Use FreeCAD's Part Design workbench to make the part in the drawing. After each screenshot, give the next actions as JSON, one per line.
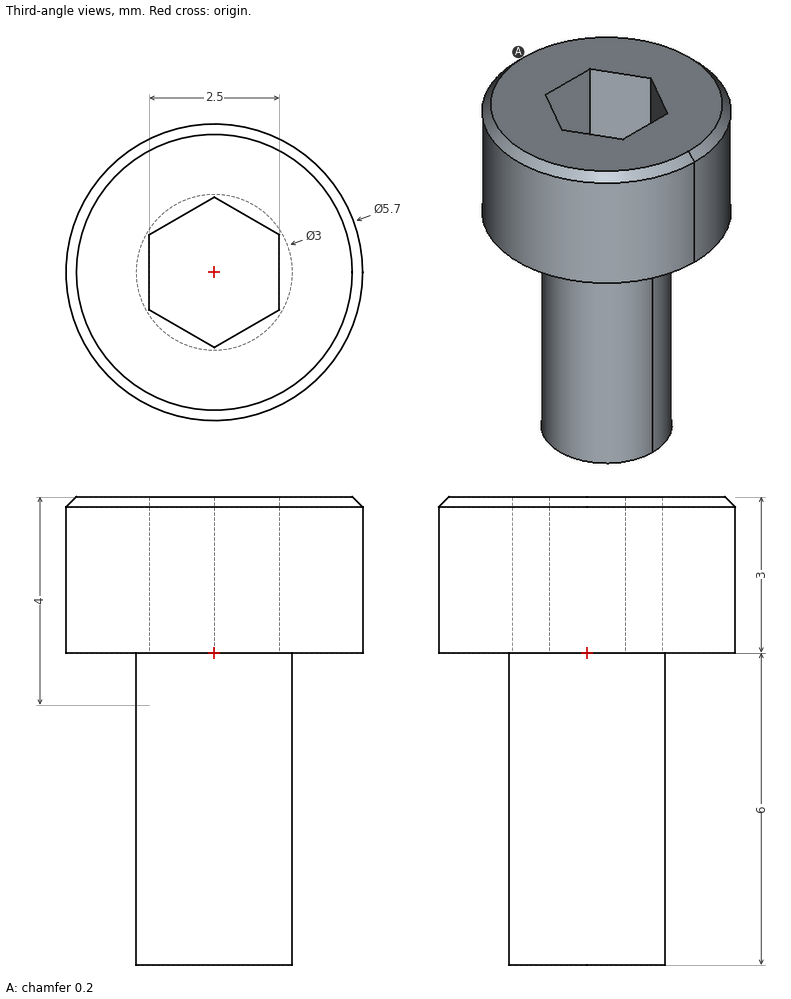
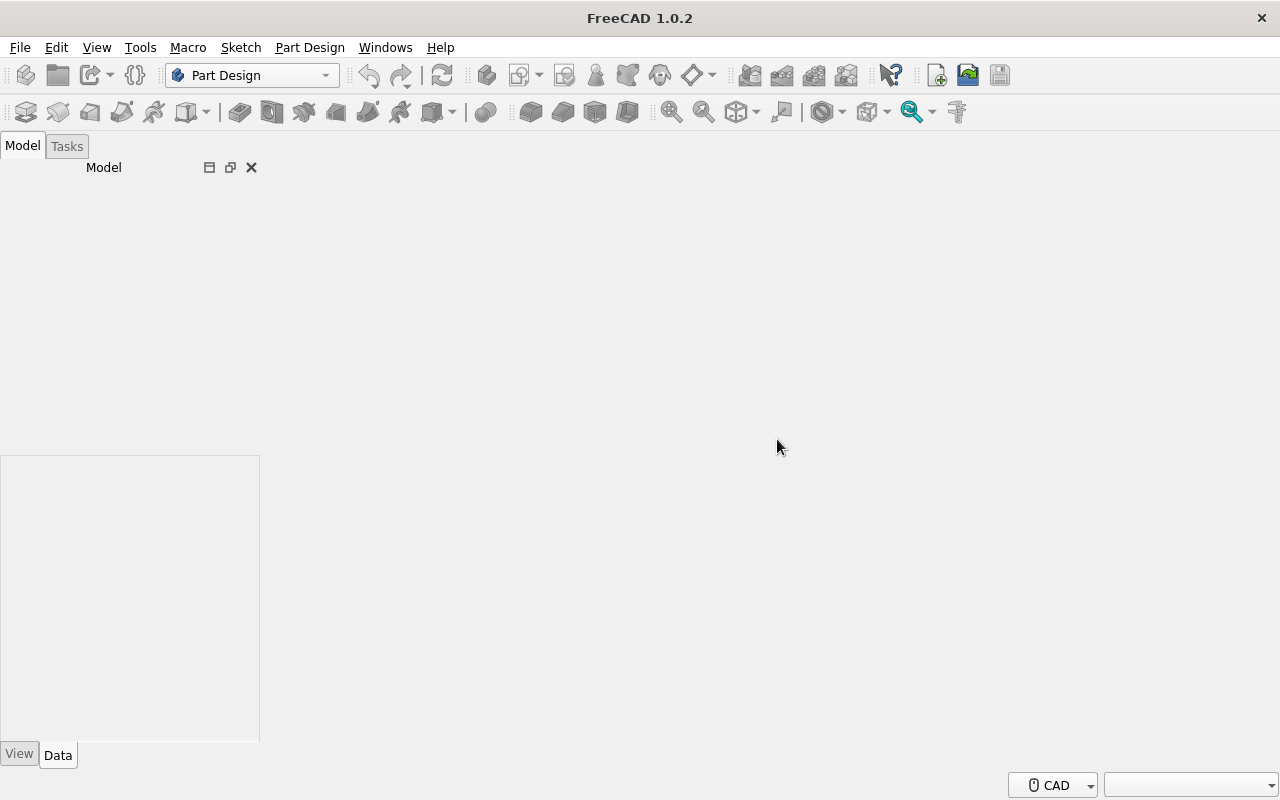
{"action": "left_click", "coordinate": [936, 76]}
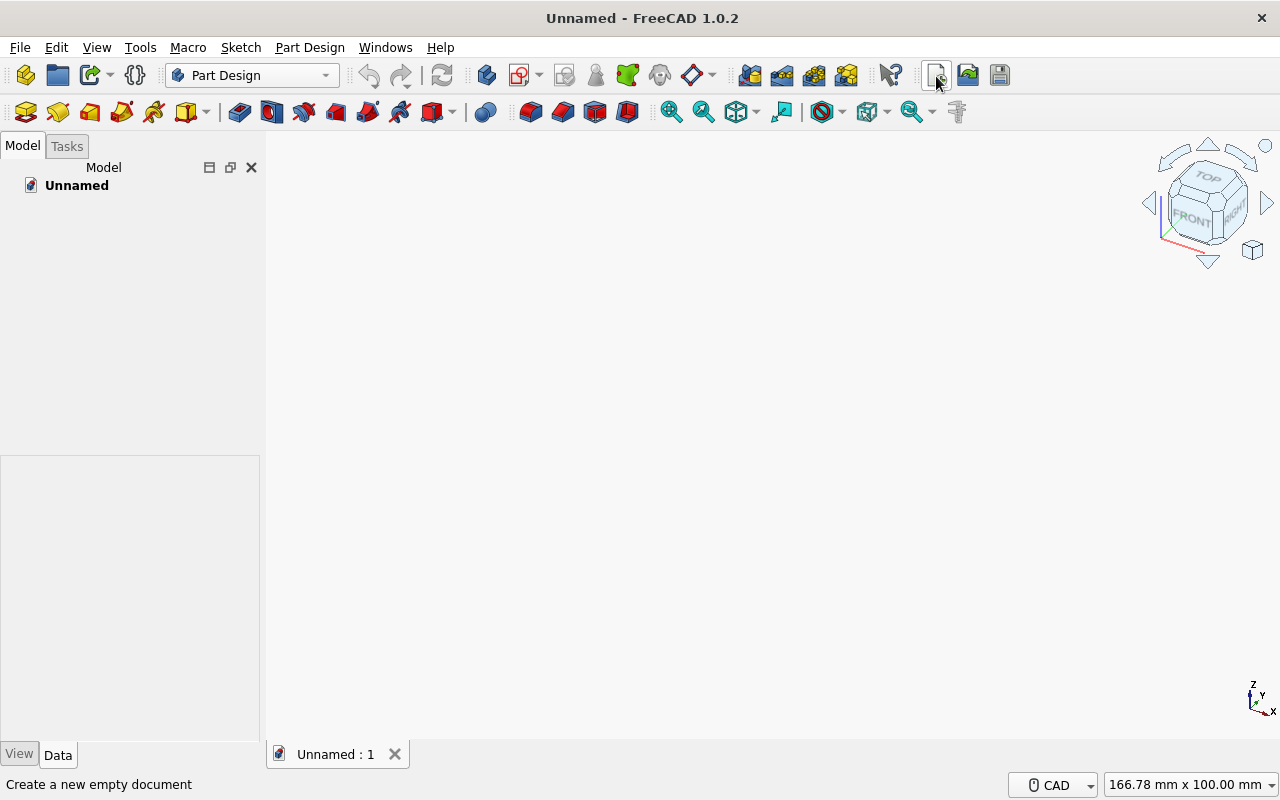
{"action": "left_click", "coordinate": [520, 76]}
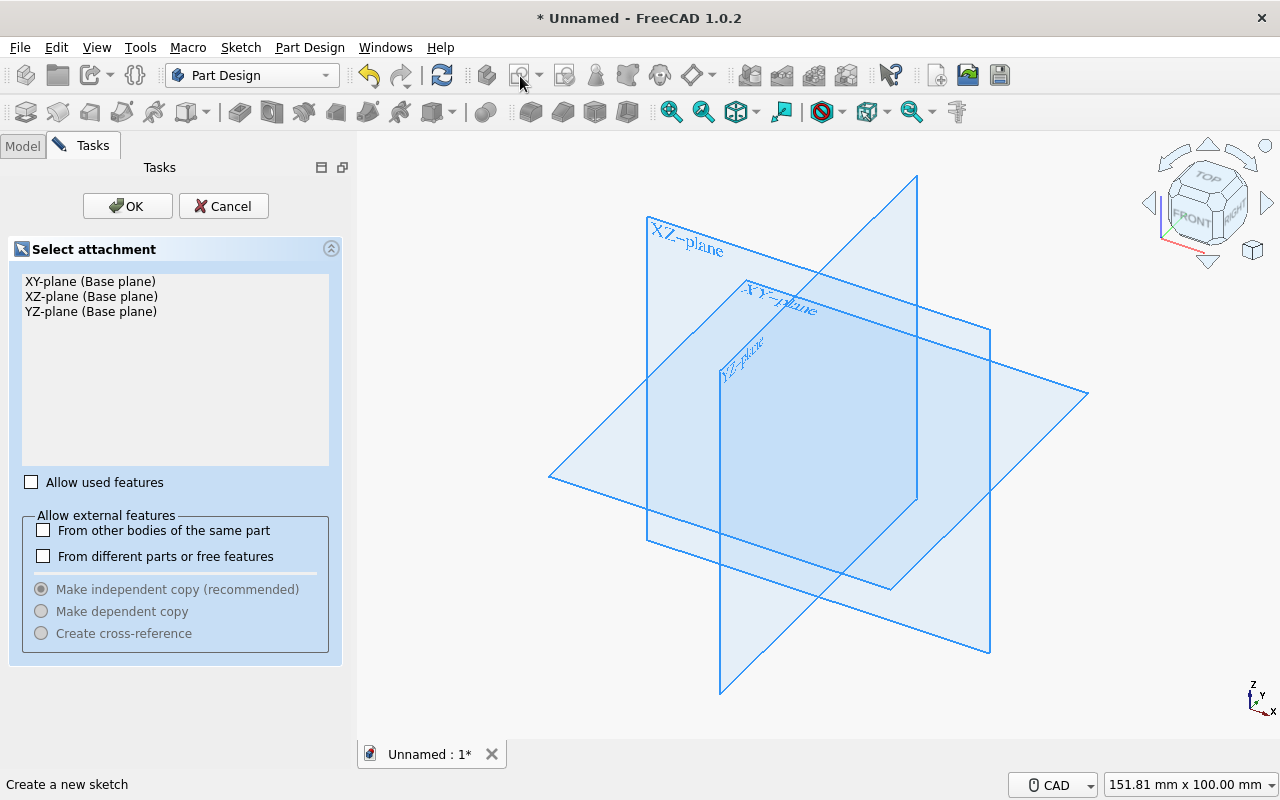
{"action": "left_click", "coordinate": [82, 282]}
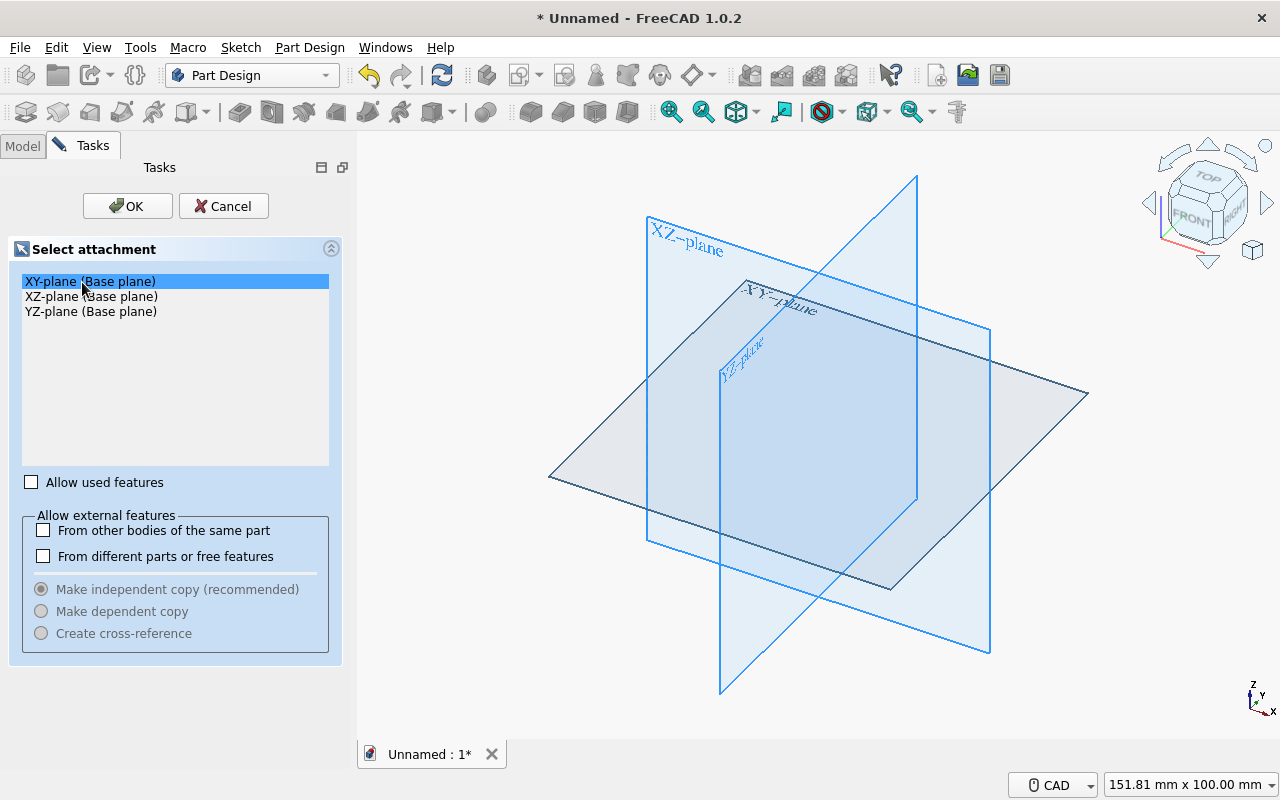
{"action": "left_click", "coordinate": [128, 206]}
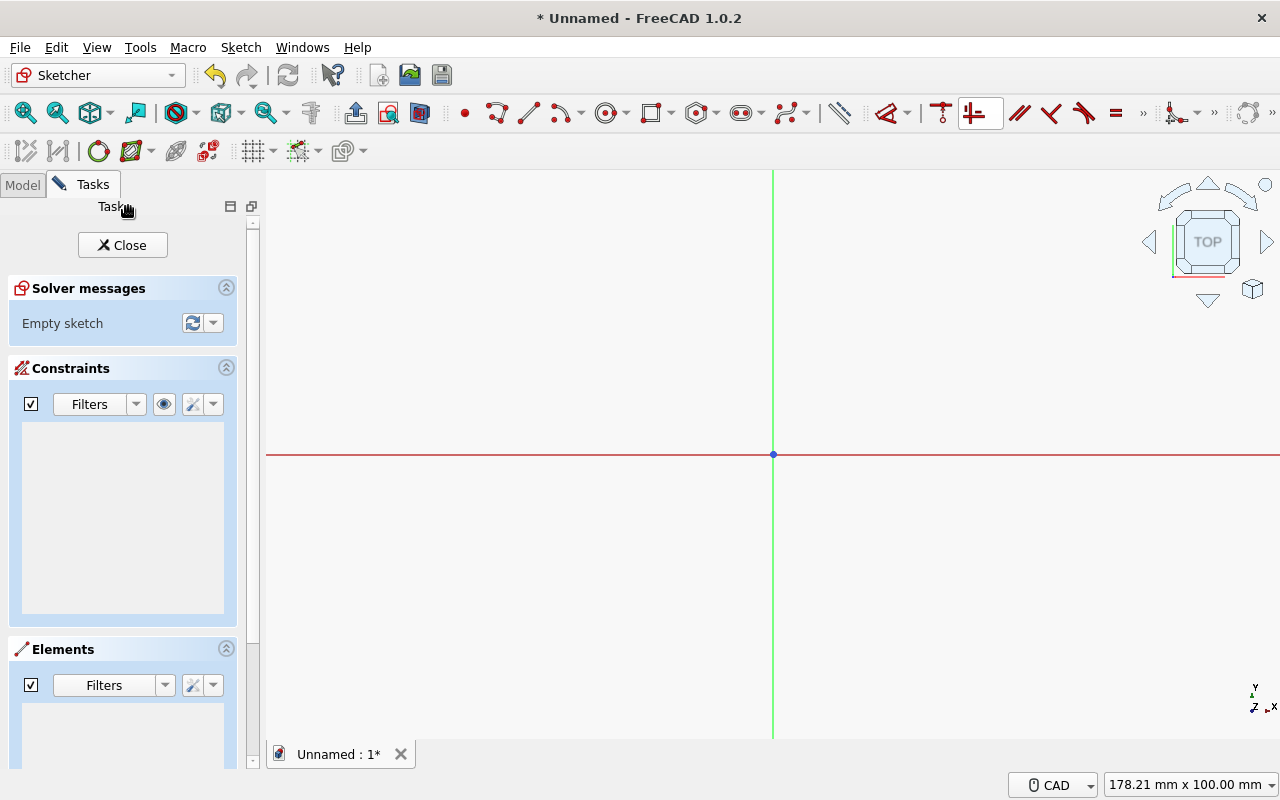
{"action": "scroll", "coordinate": [780, 455], "scroll_direction": "up", "scroll_amount": 12}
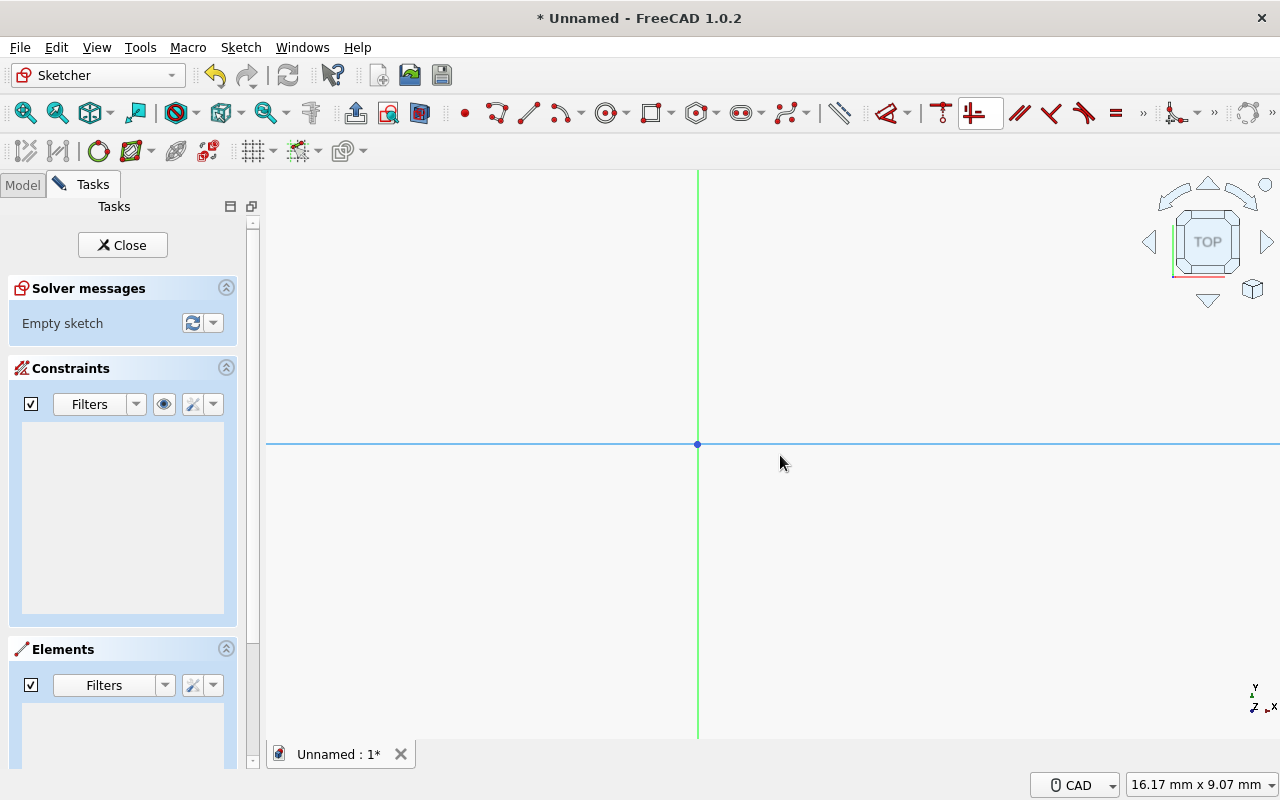
{"action": "key", "text": "g c"}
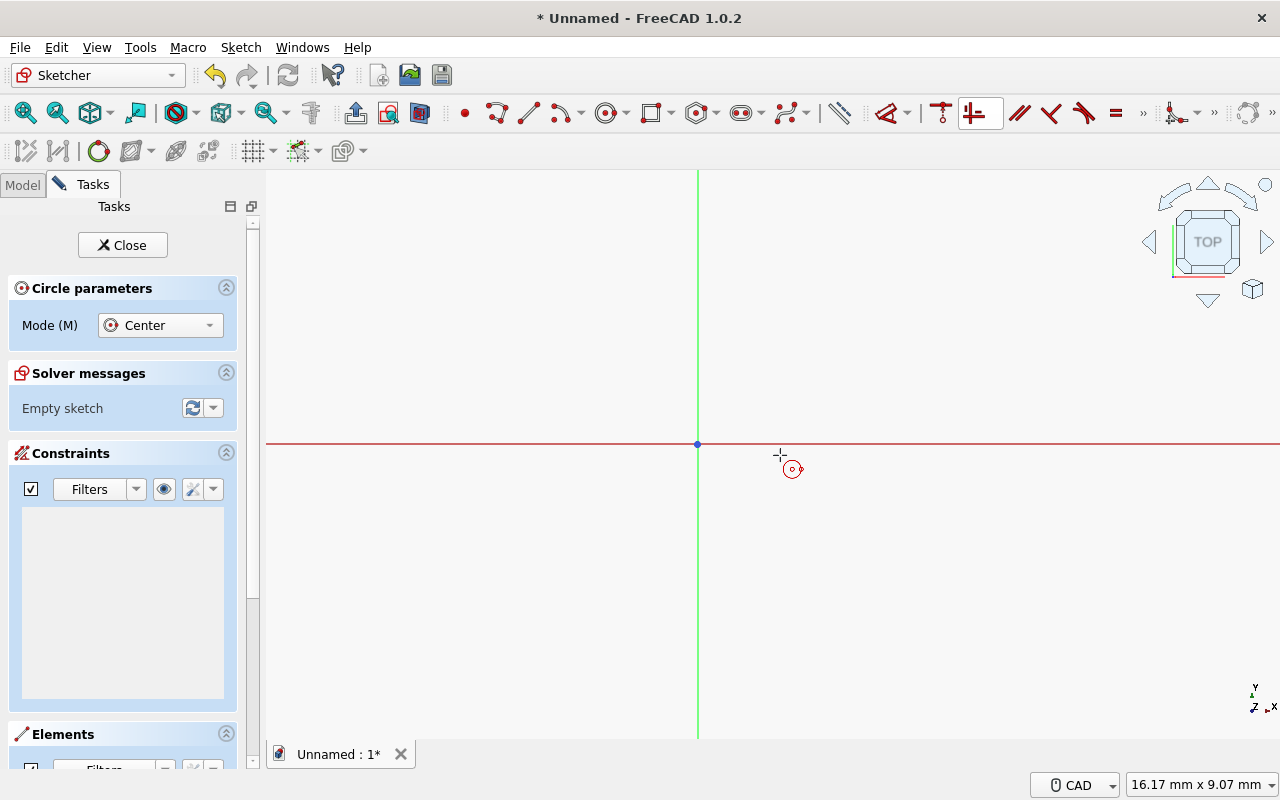
{"action": "left_click", "coordinate": [698, 444]}
{"action": "left_click", "coordinate": [824, 318]}
{"action": "key", "text": "Escape"}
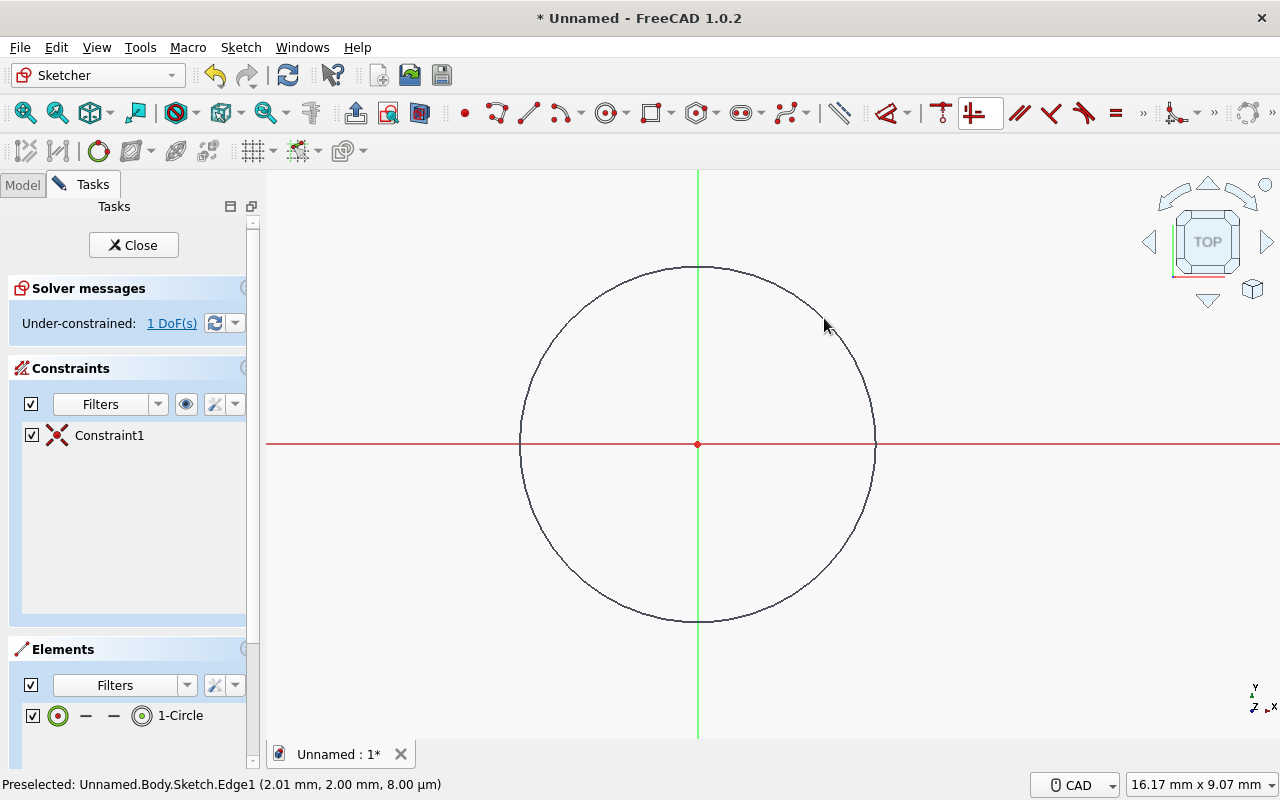
{"action": "key", "text": "d"}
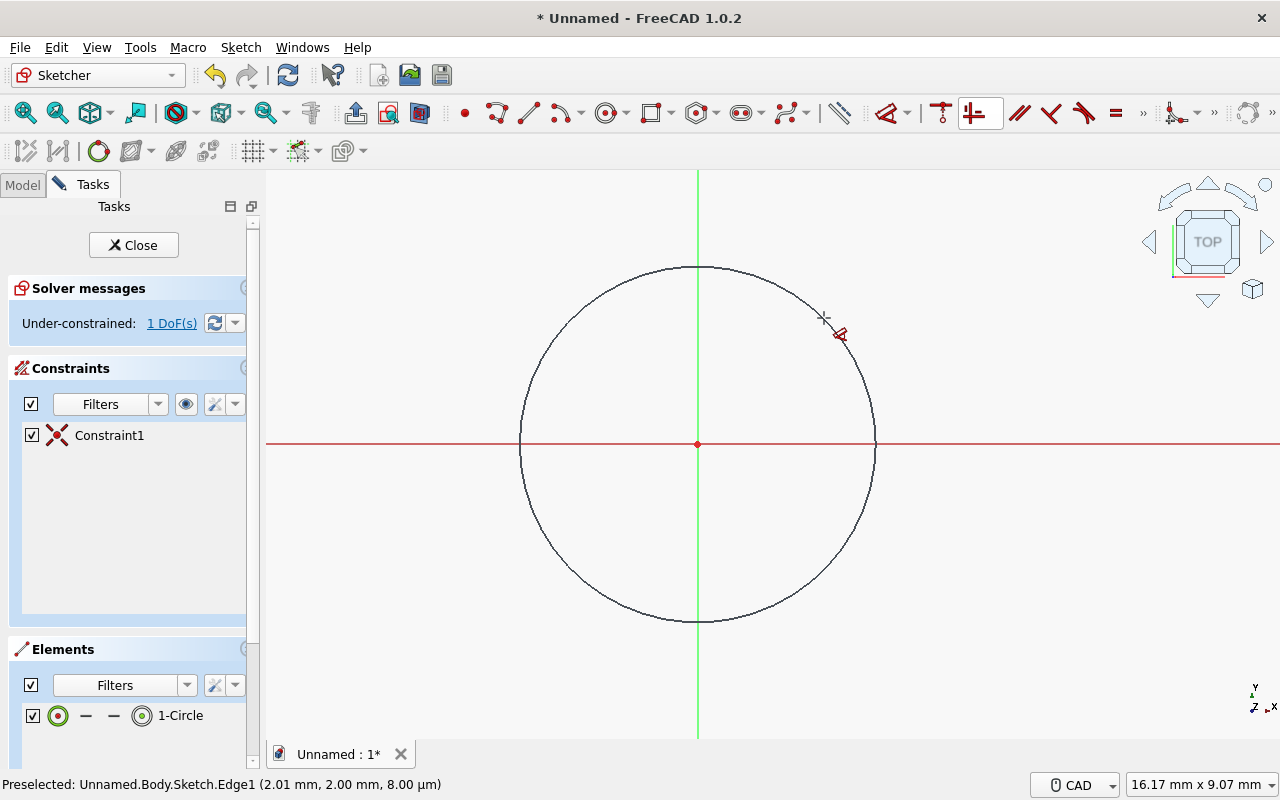
{"action": "left_click", "coordinate": [823, 318]}
{"action": "left_click", "coordinate": [846, 295]}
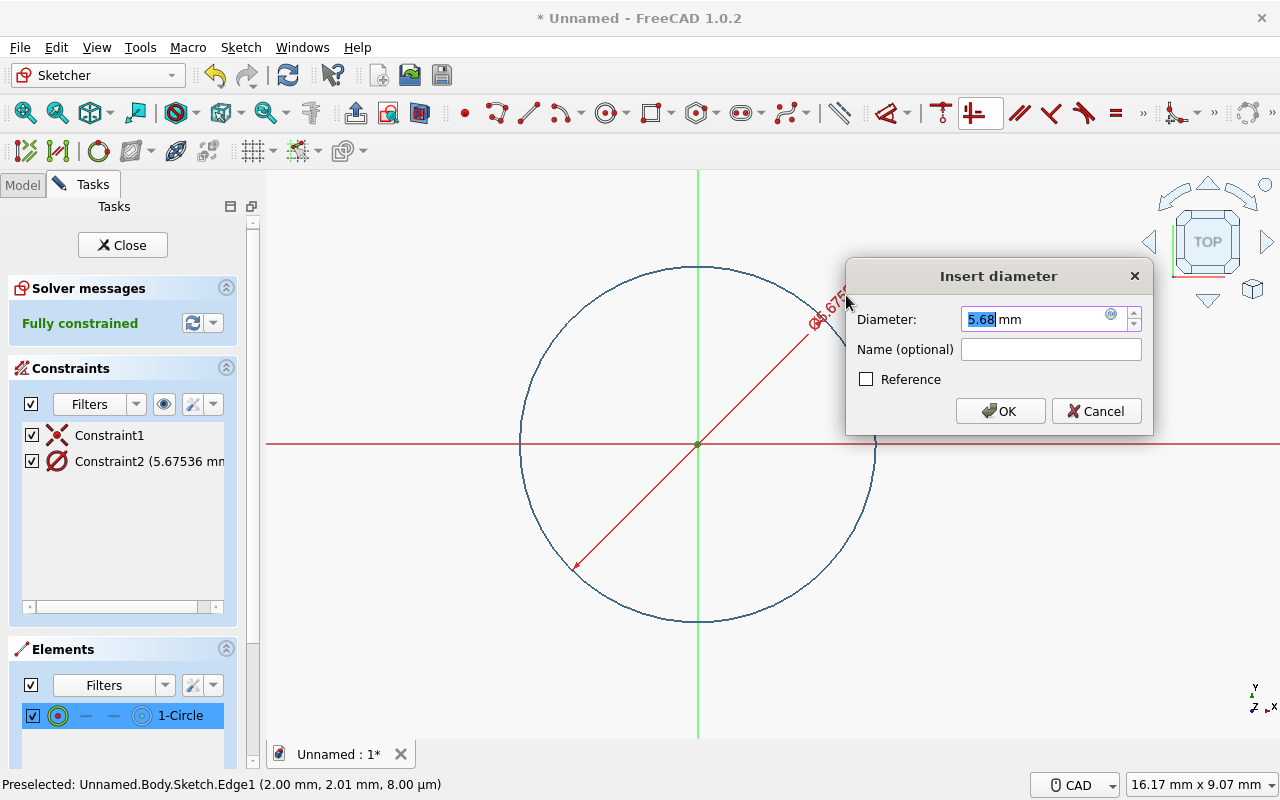
{"action": "type", "text": "5.7"}
{"action": "key", "text": "Return"}
{"action": "key", "text": "Escape"}